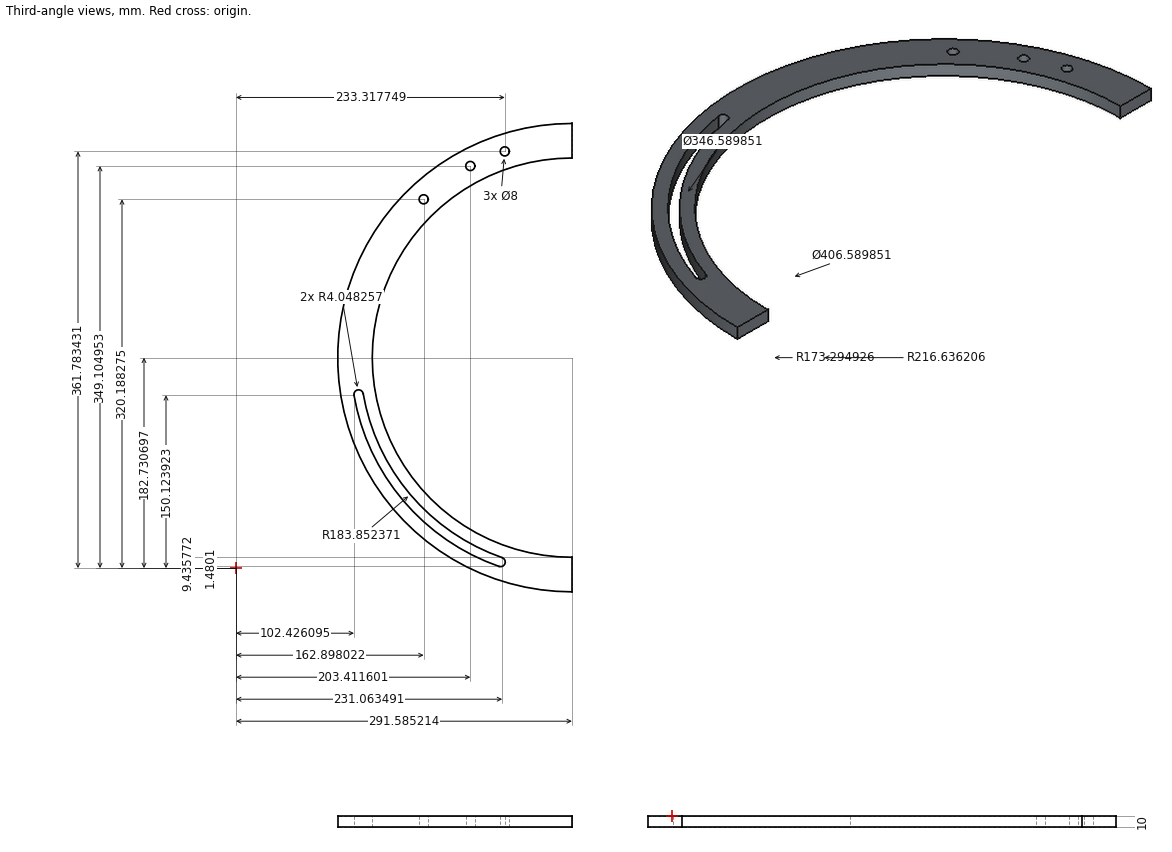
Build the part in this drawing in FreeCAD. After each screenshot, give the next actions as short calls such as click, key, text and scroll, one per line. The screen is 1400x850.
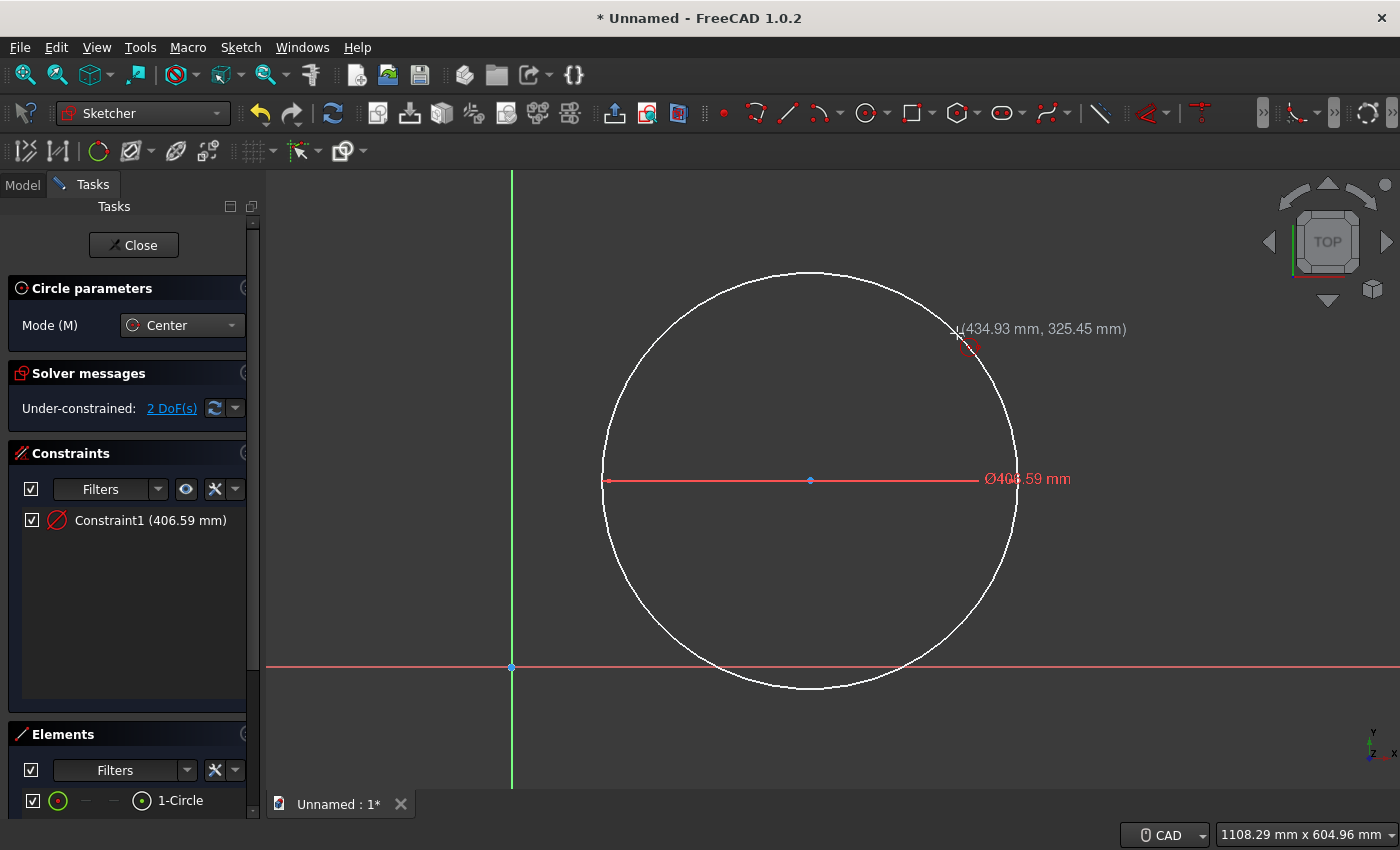
click(810, 481)
move(936, 355)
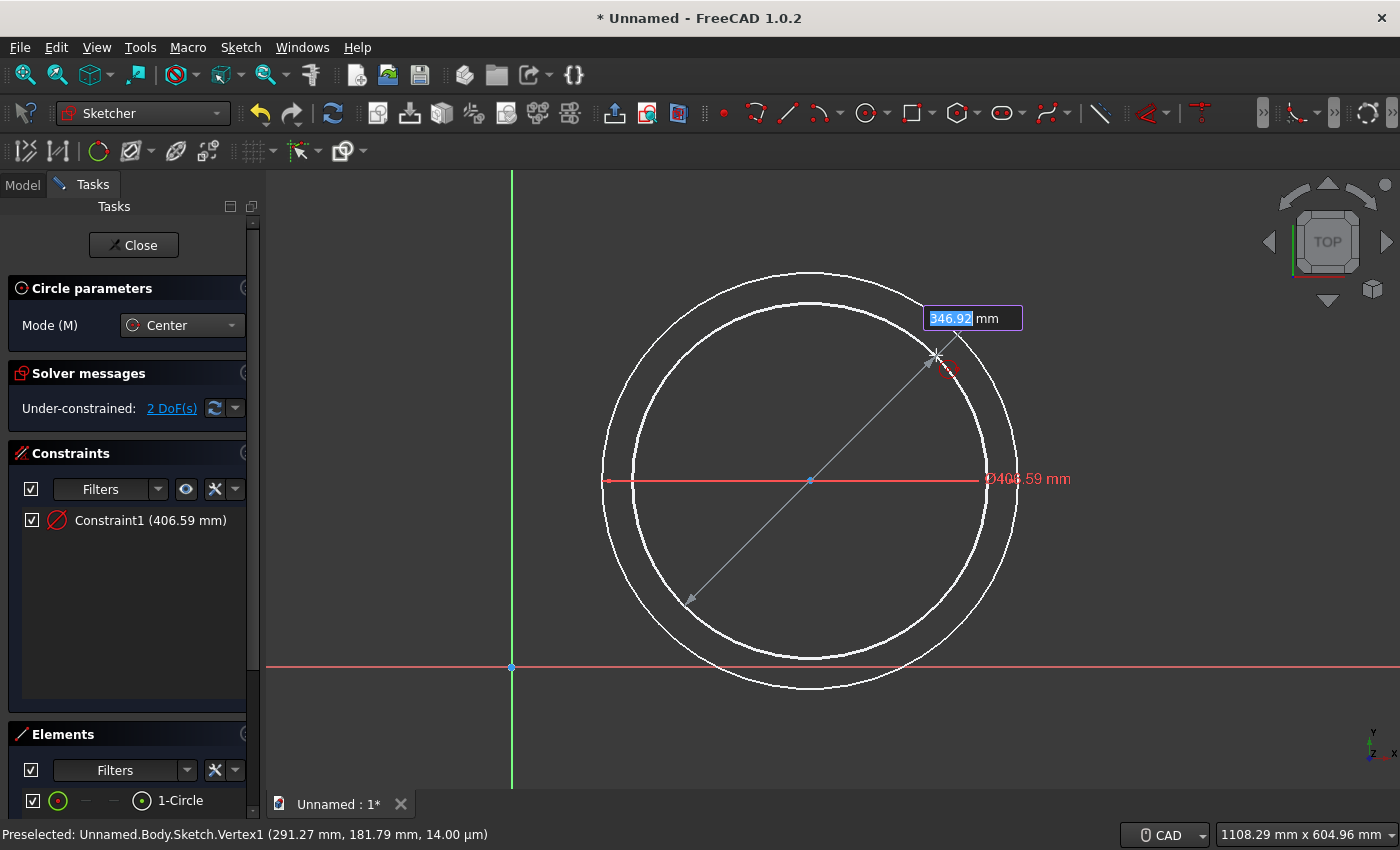
text(346.589851)
key(Return)
key(Escape)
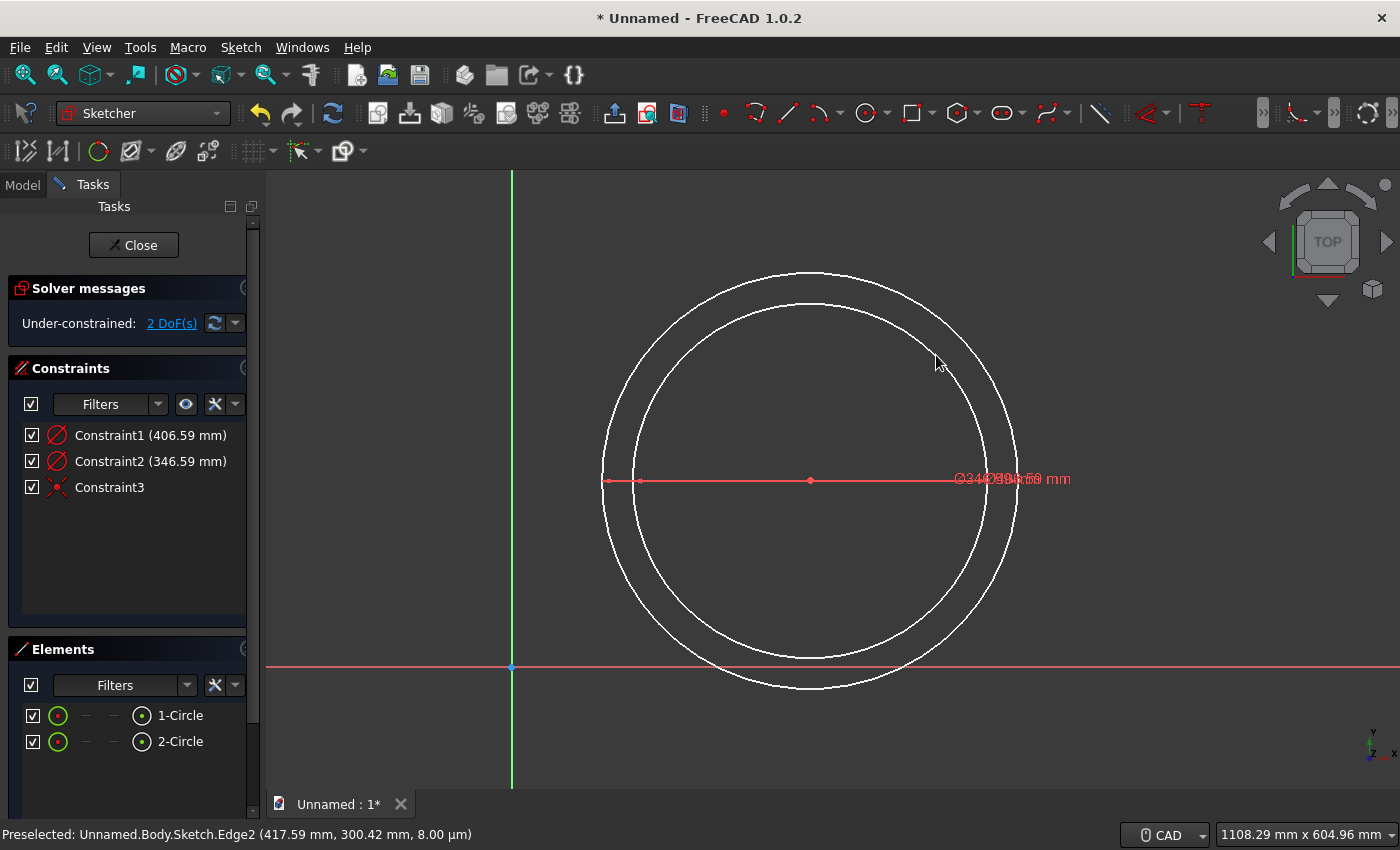
key(d)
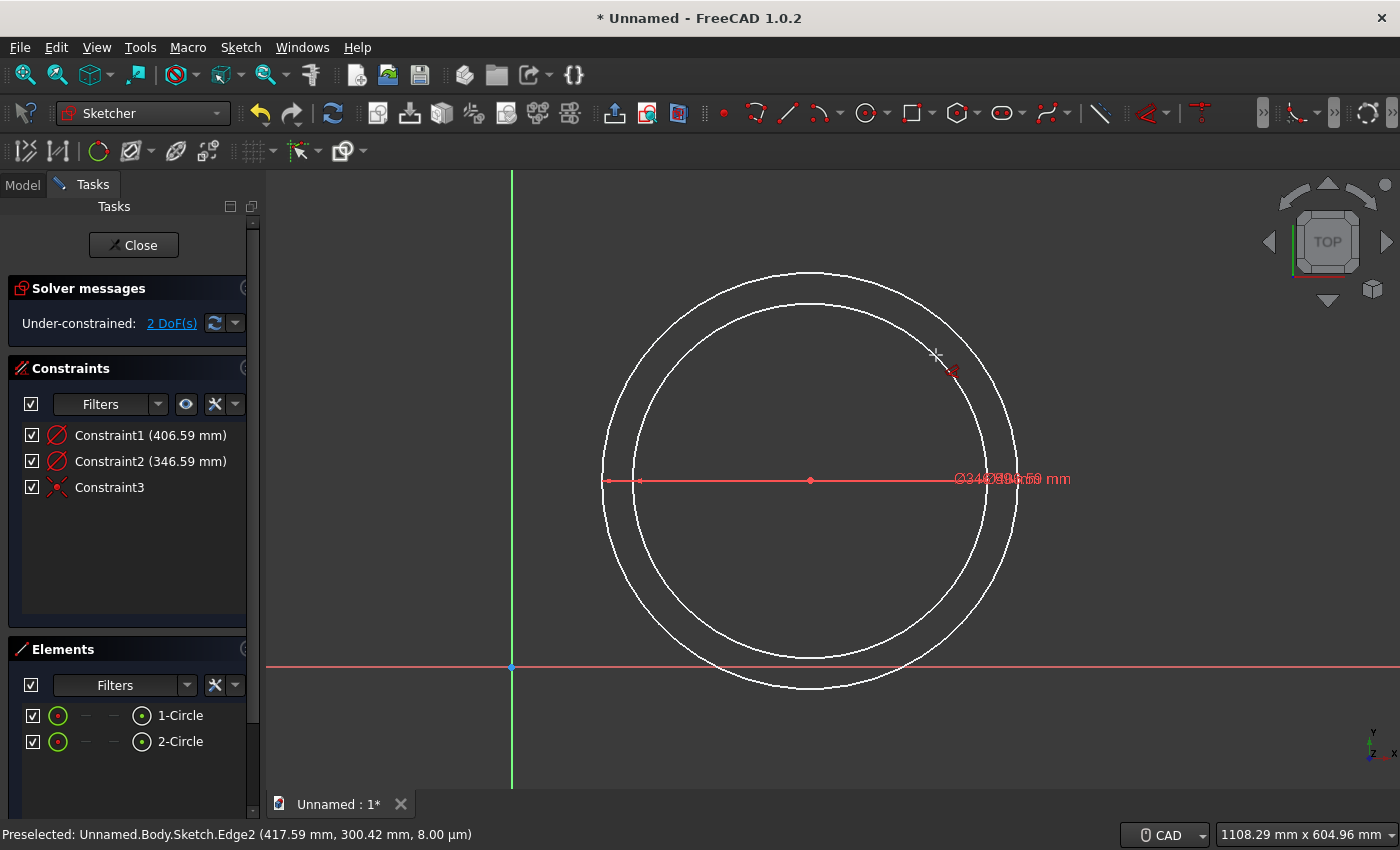
click(810, 481)
click(661, 701)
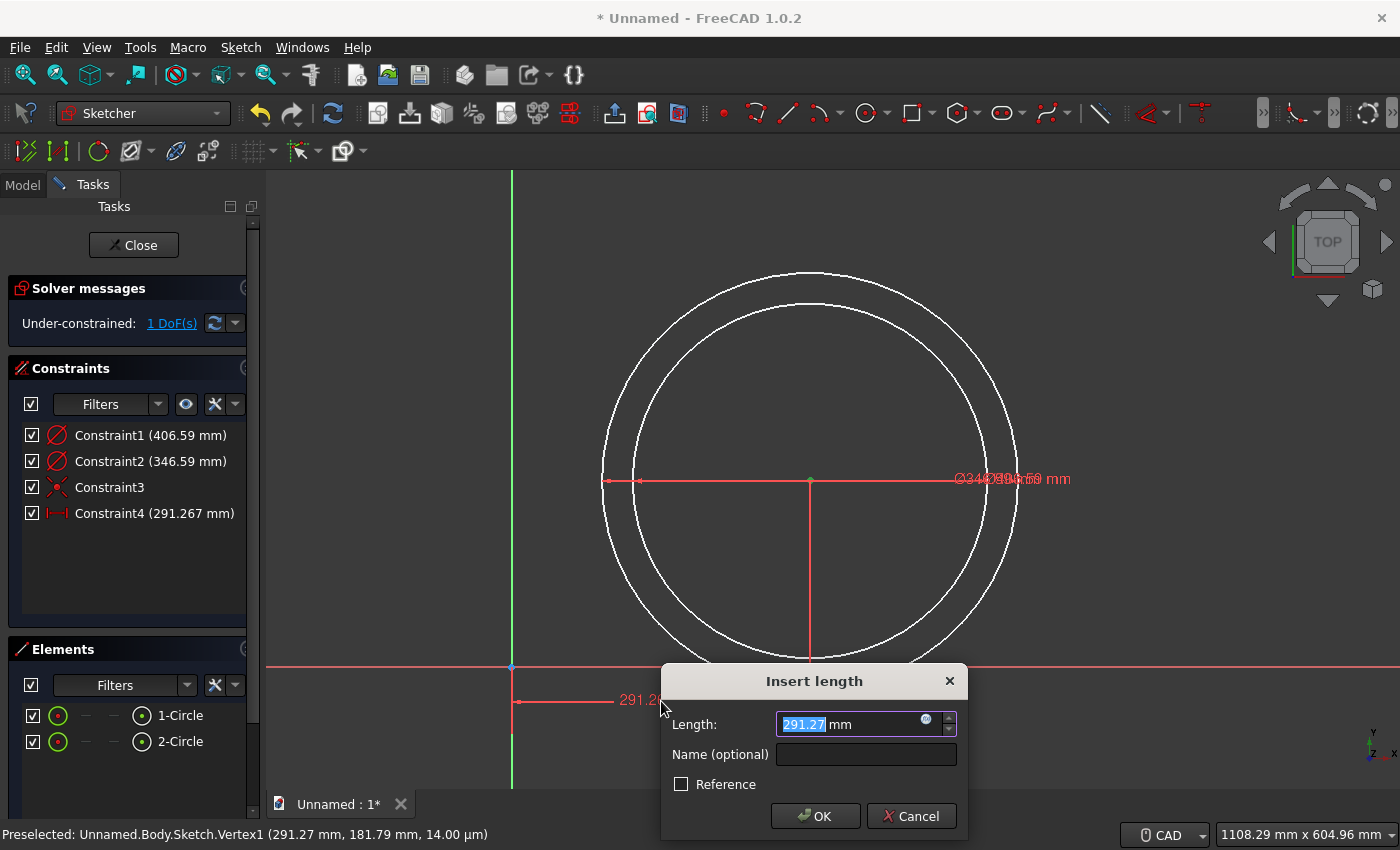
text(291.585214)
key(Return)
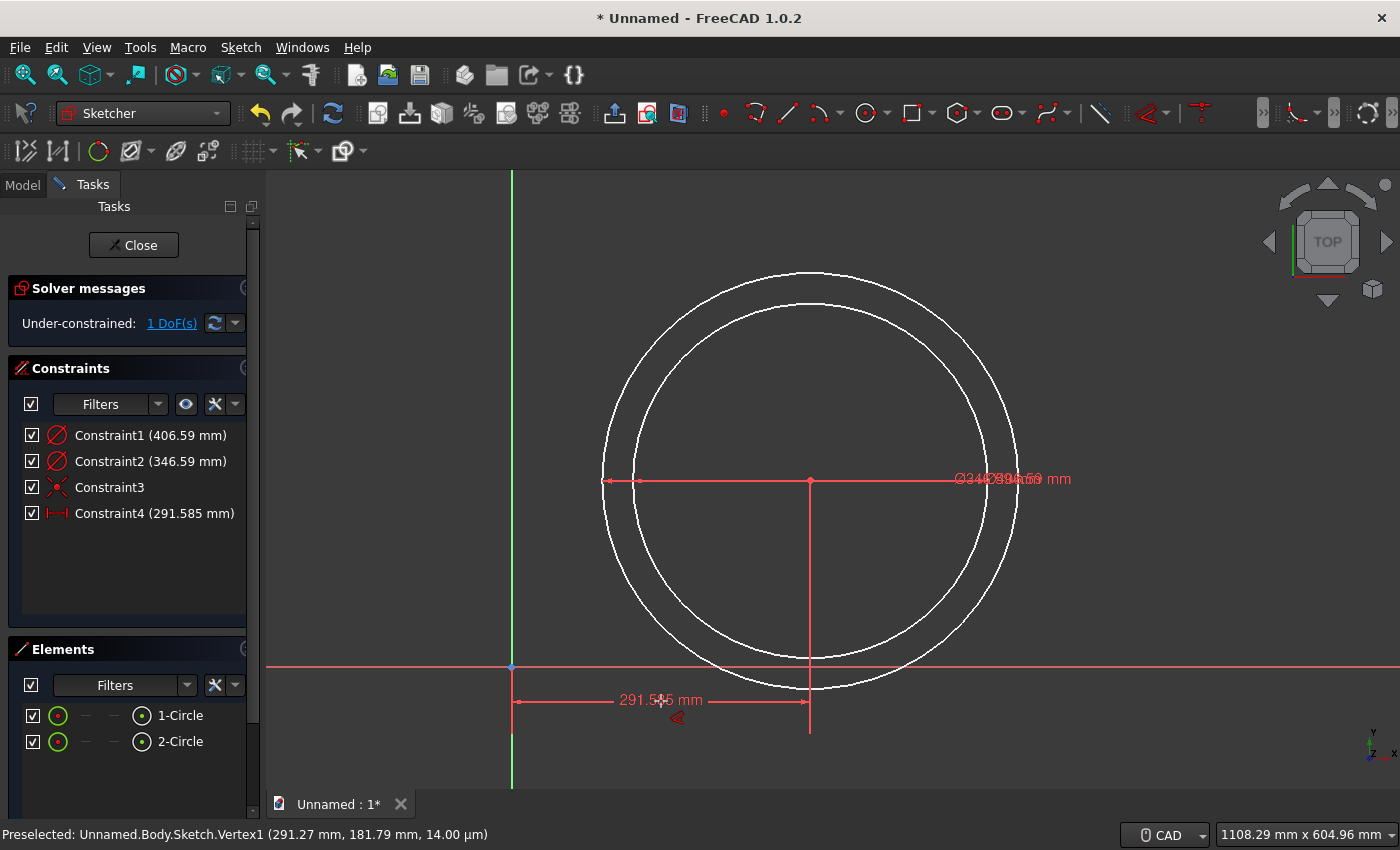
click(810, 481)
click(478, 574)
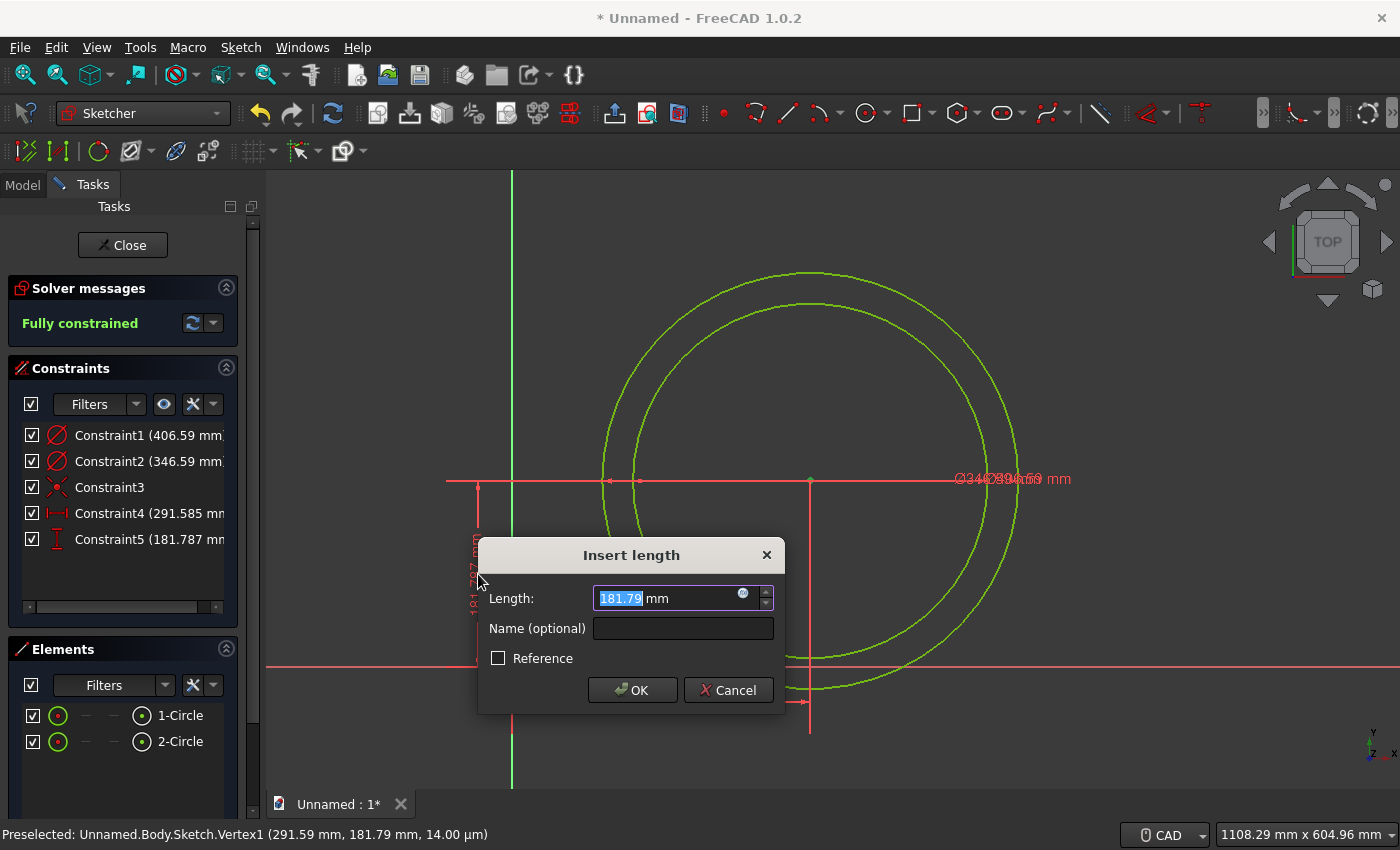
text(182.730697)
key(Return)
key(Escape)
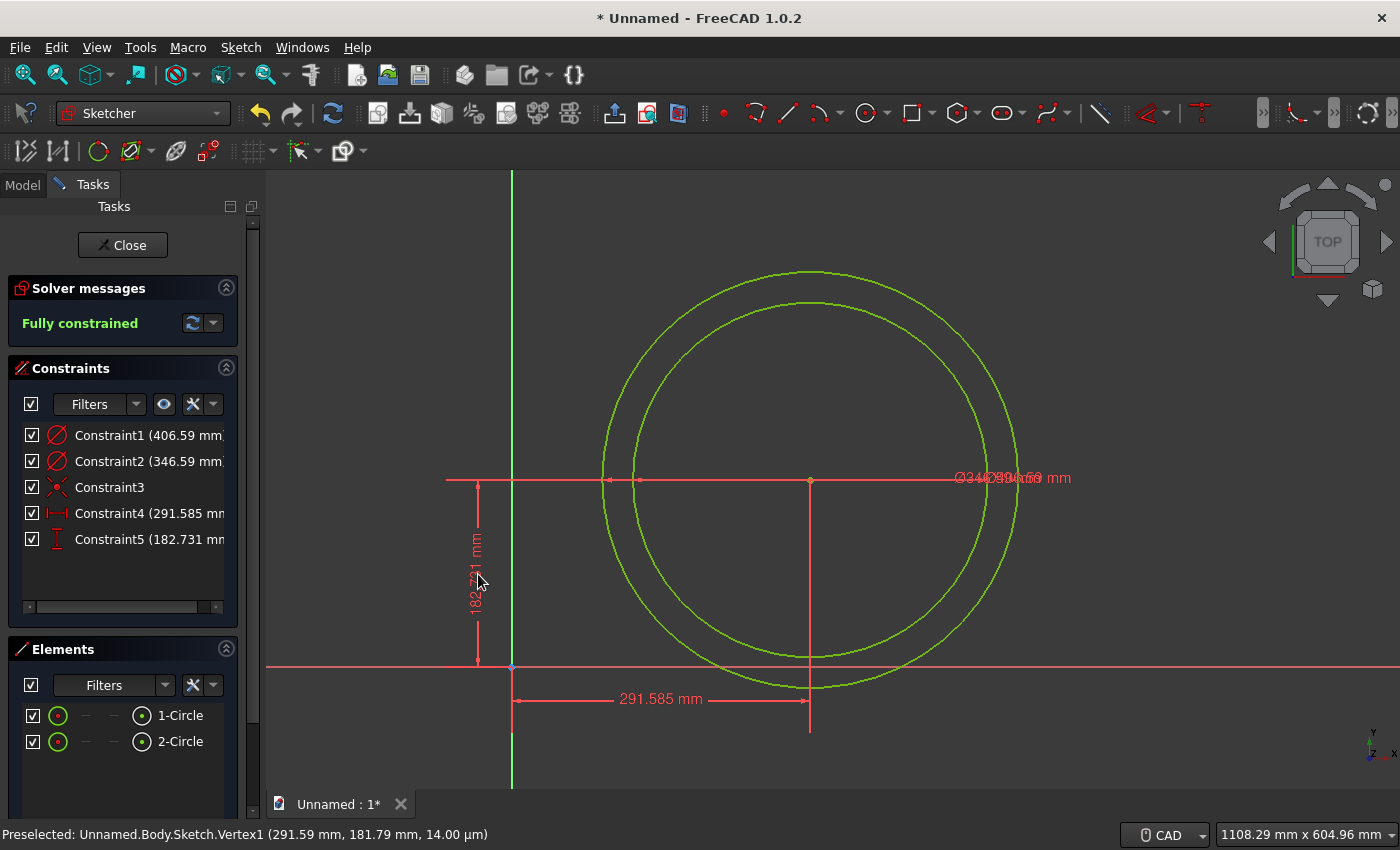
click(123, 245)